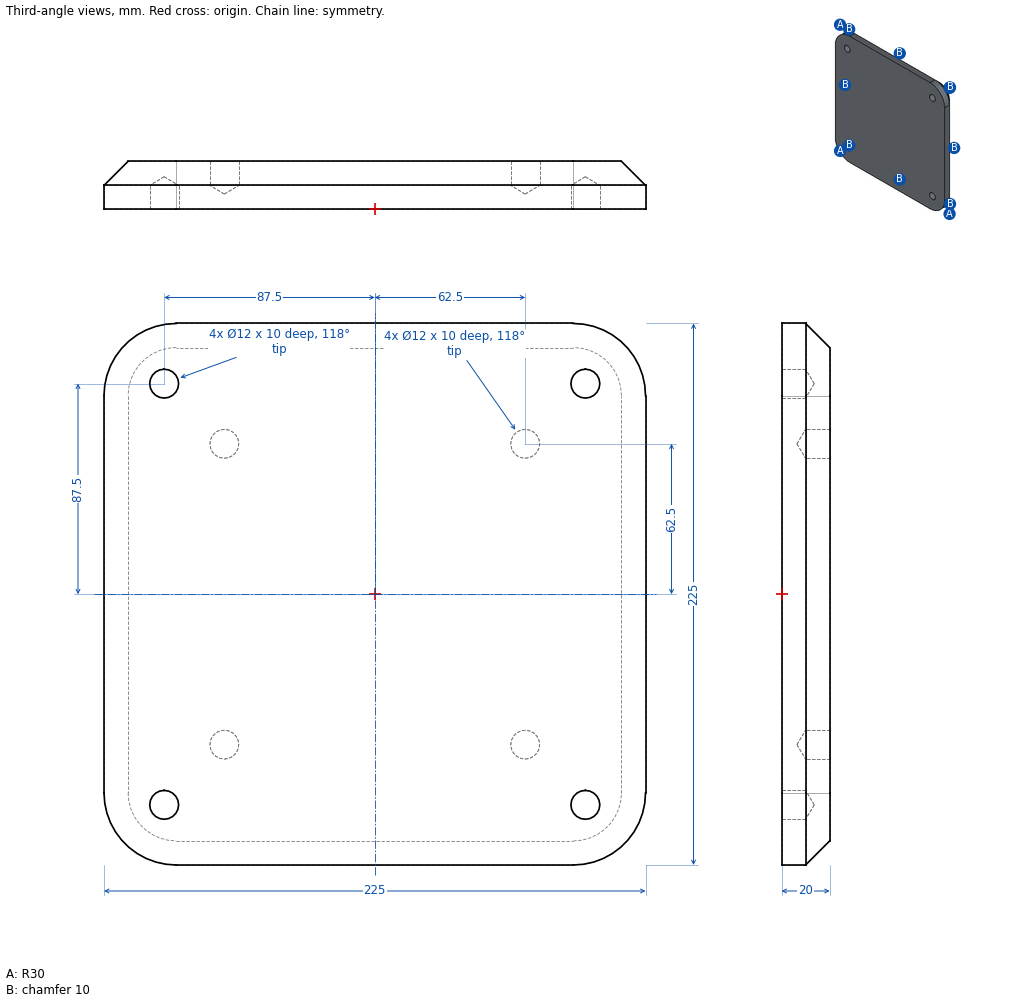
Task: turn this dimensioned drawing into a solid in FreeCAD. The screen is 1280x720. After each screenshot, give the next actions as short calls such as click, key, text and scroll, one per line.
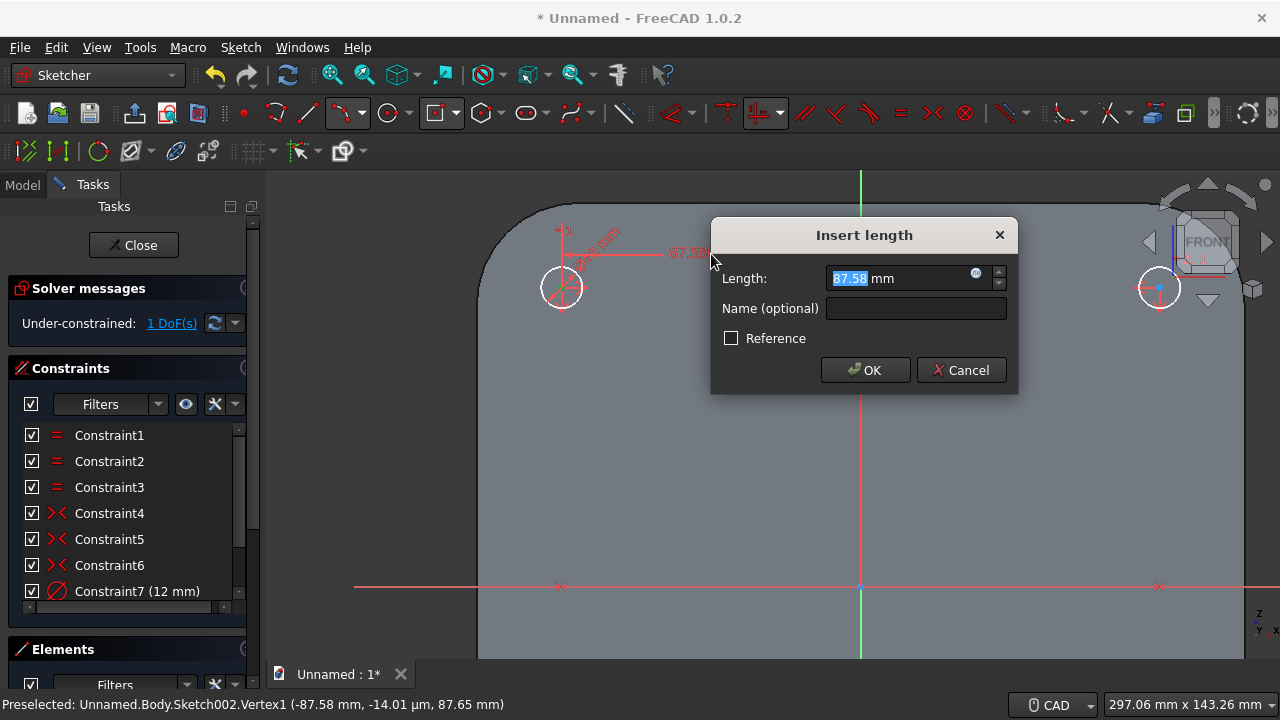
text(87.5)
key(Return)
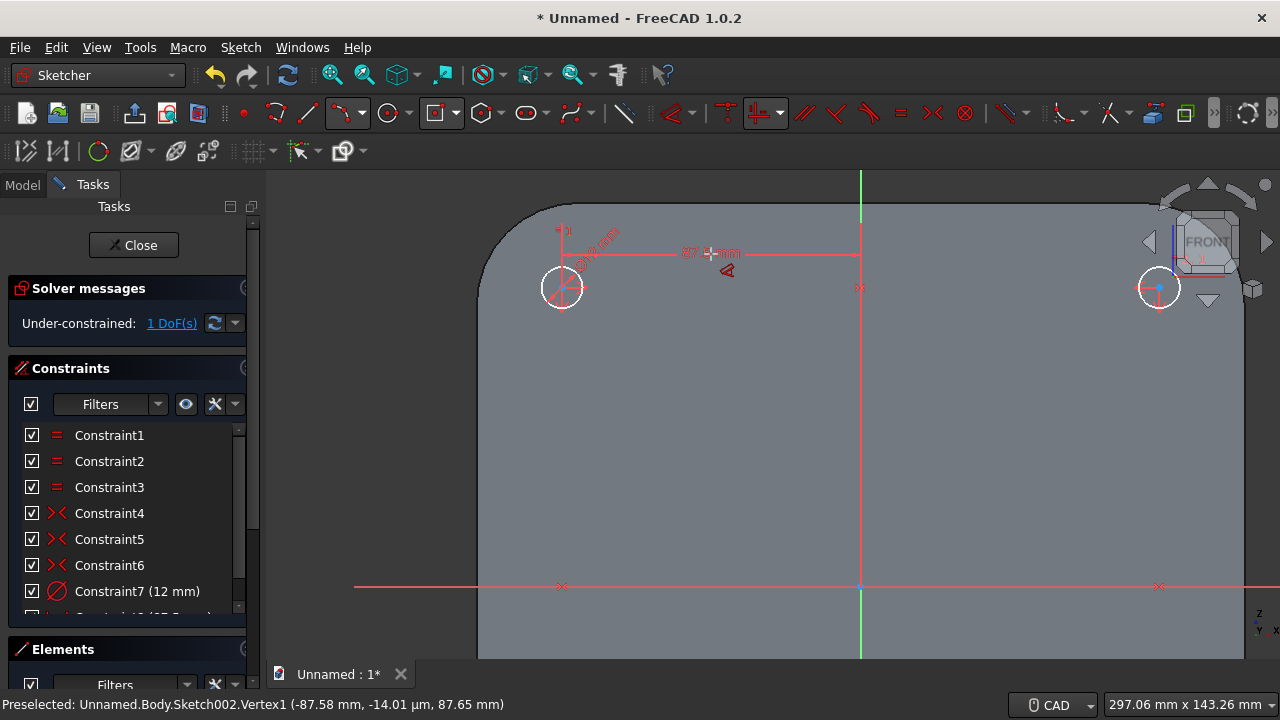
click(562, 288)
click(528, 437)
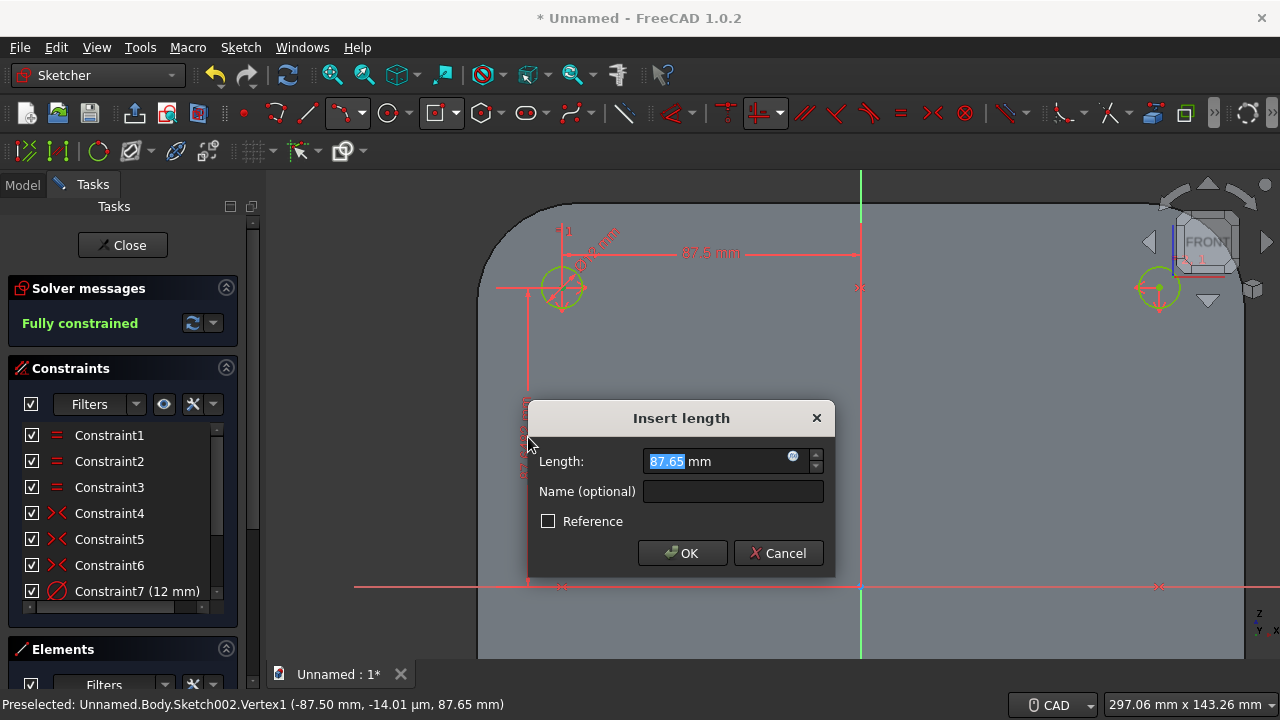
text(87.5)
key(Return)
key(Escape)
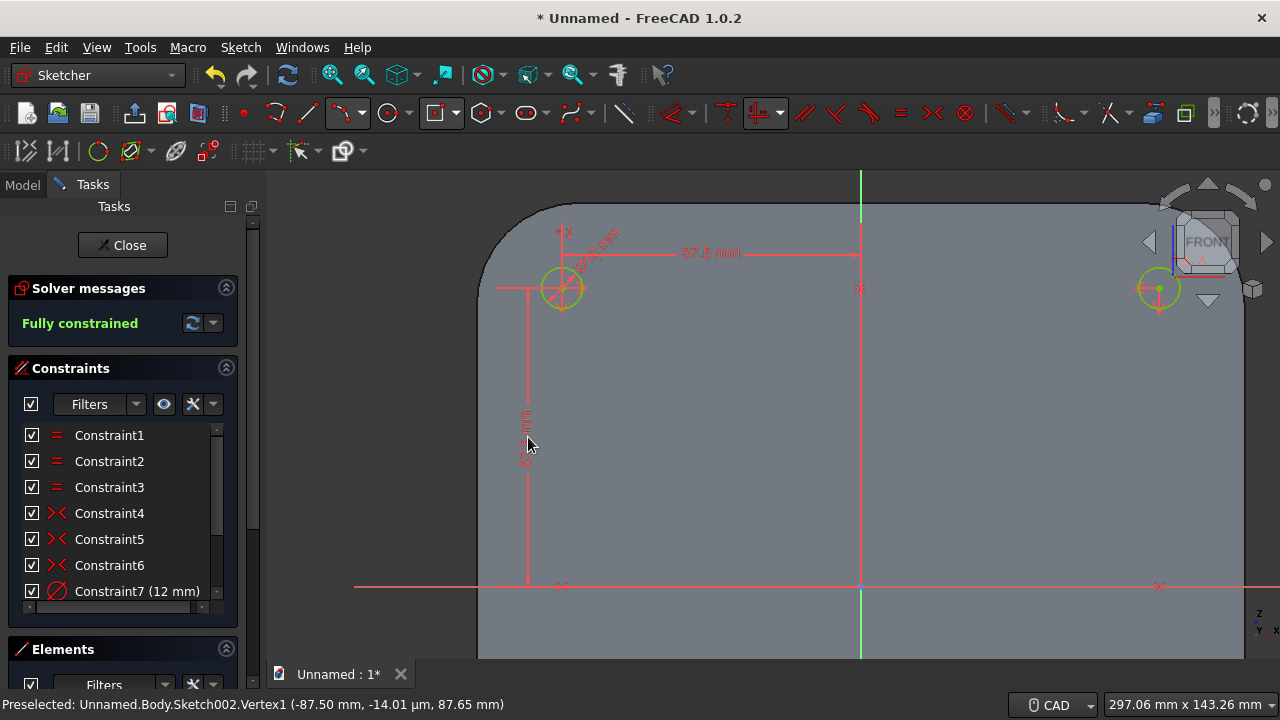
click(123, 245)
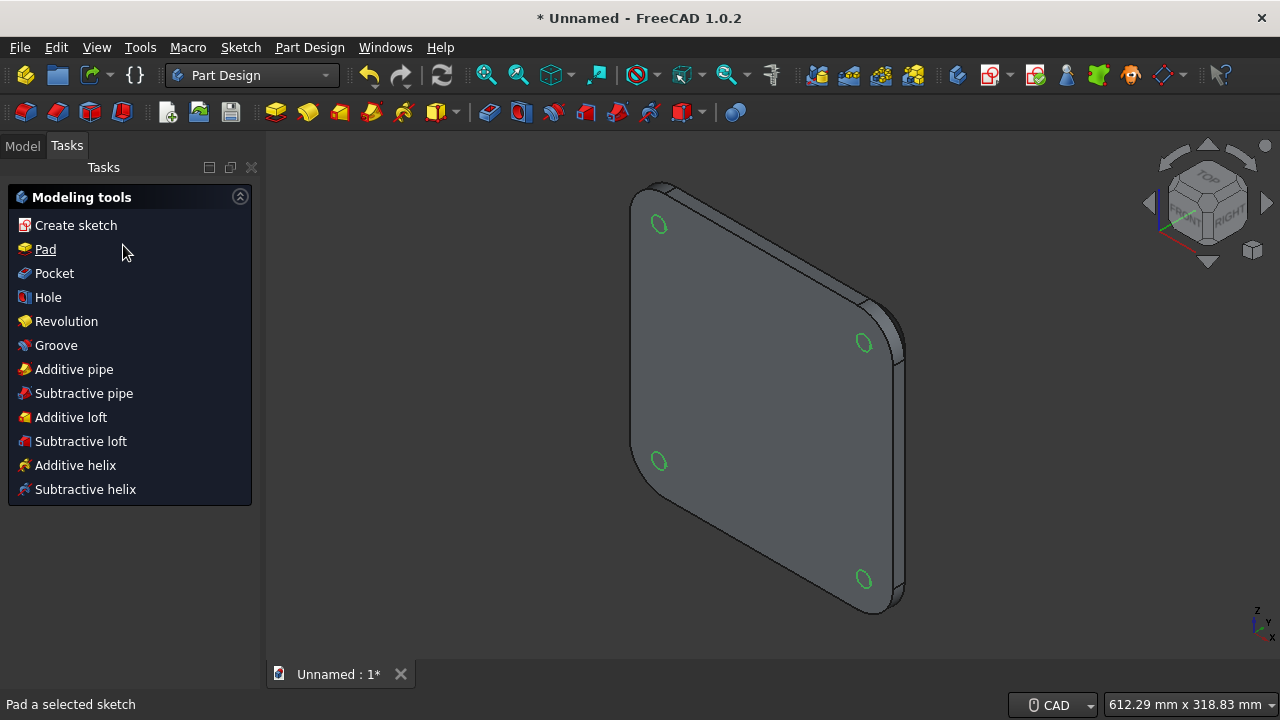
click(522, 112)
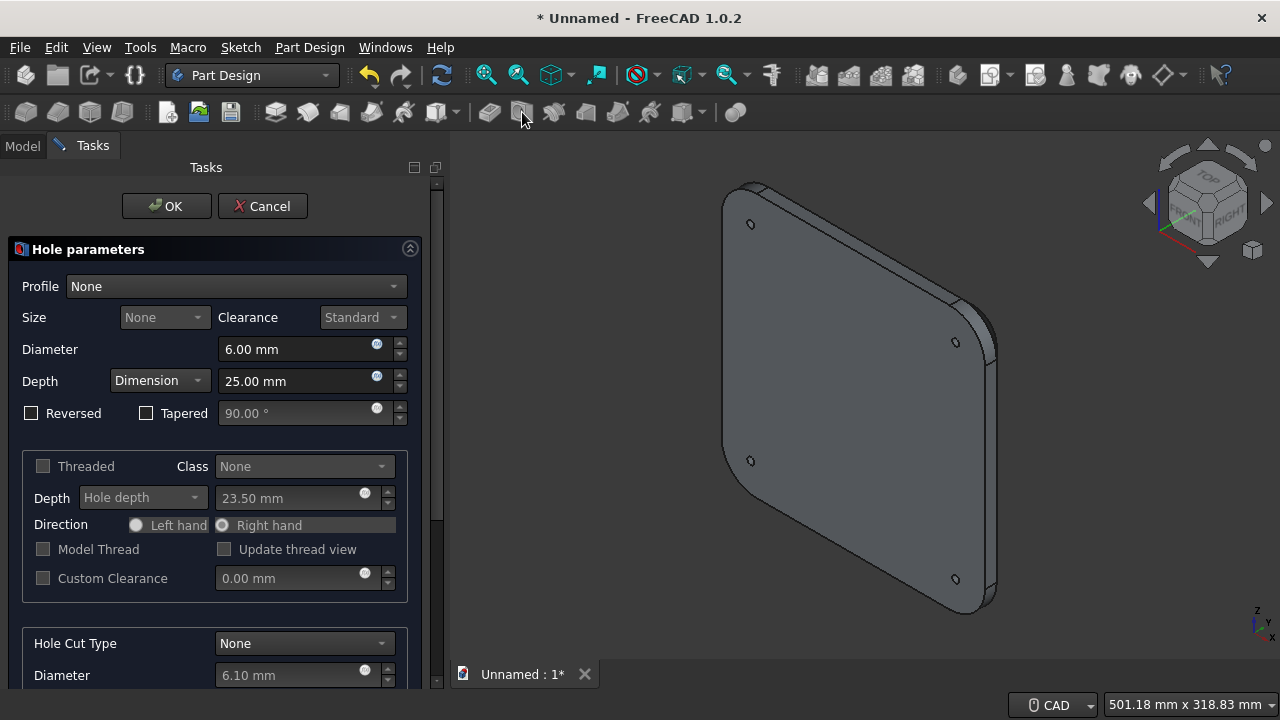
triple_click(305, 349)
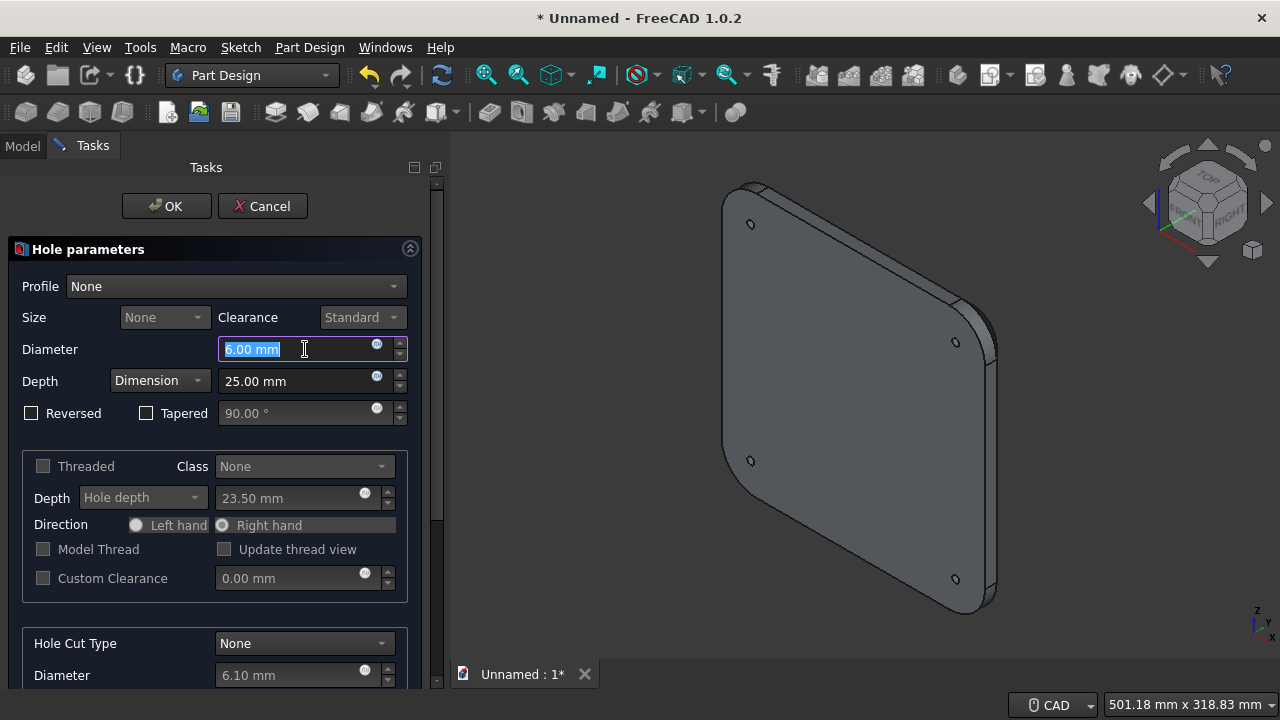
text(12)
key(Tab)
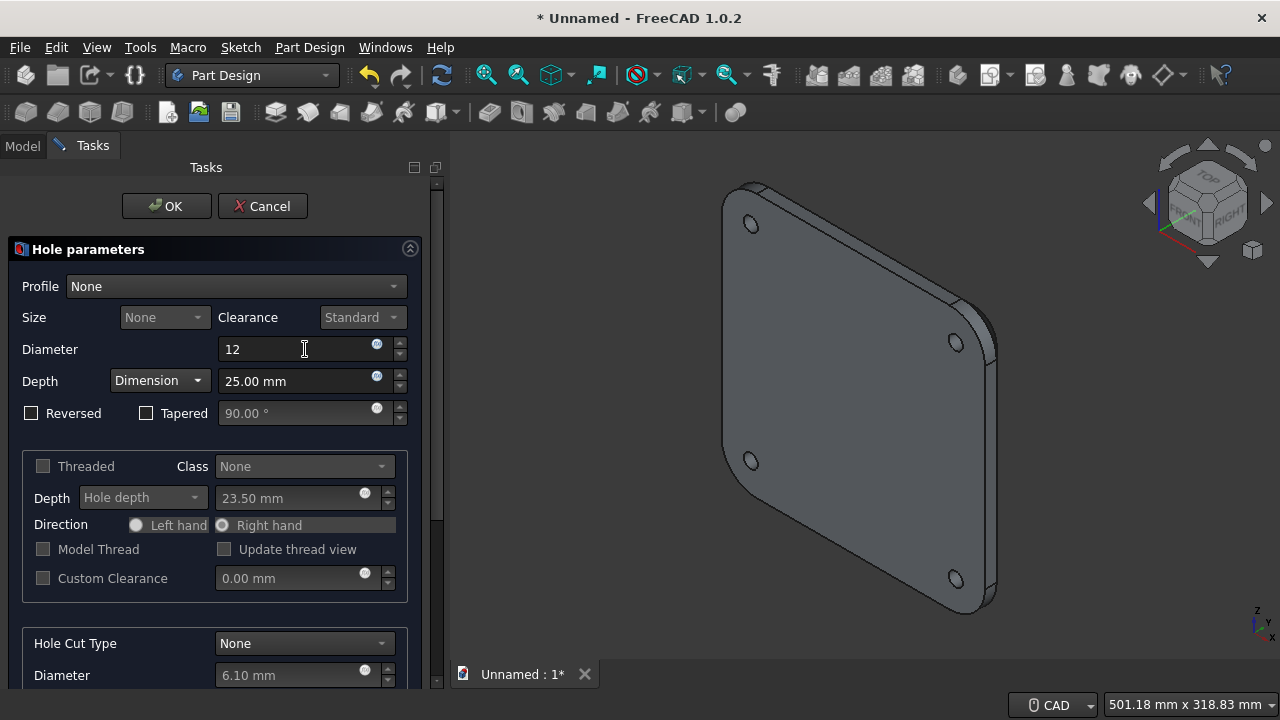
triple_click(305, 381)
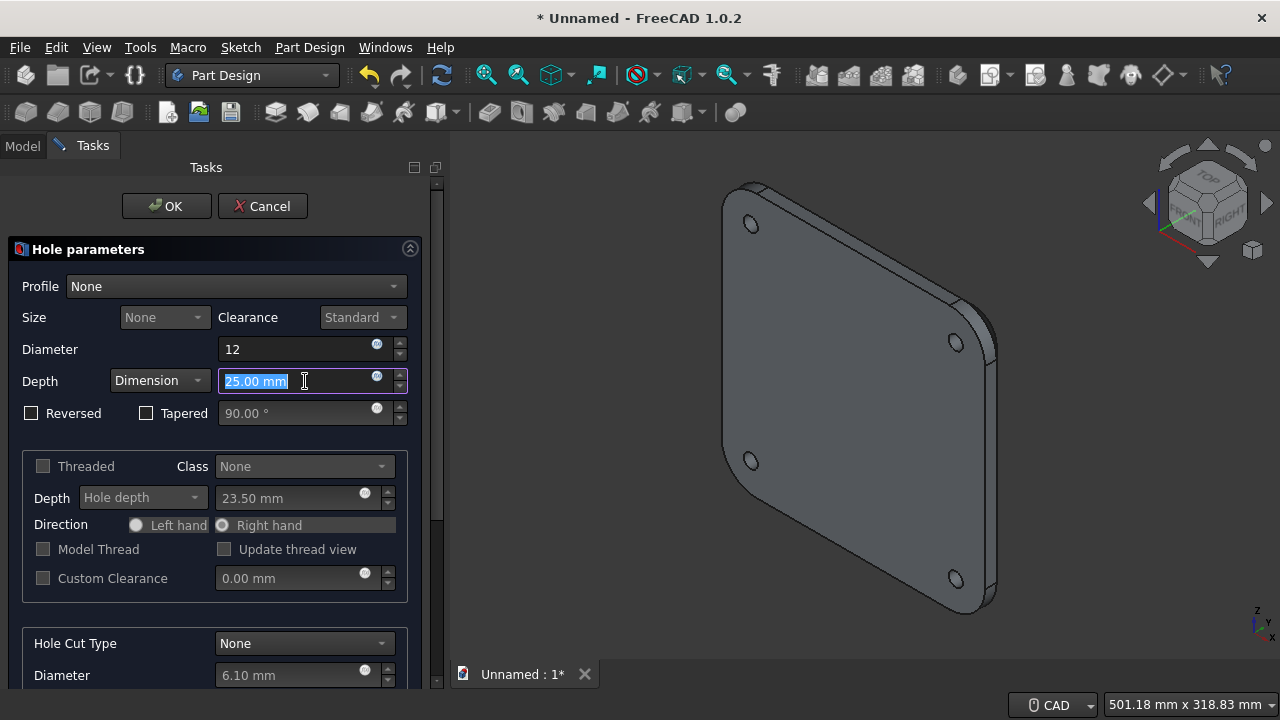
text(10)
key(Tab)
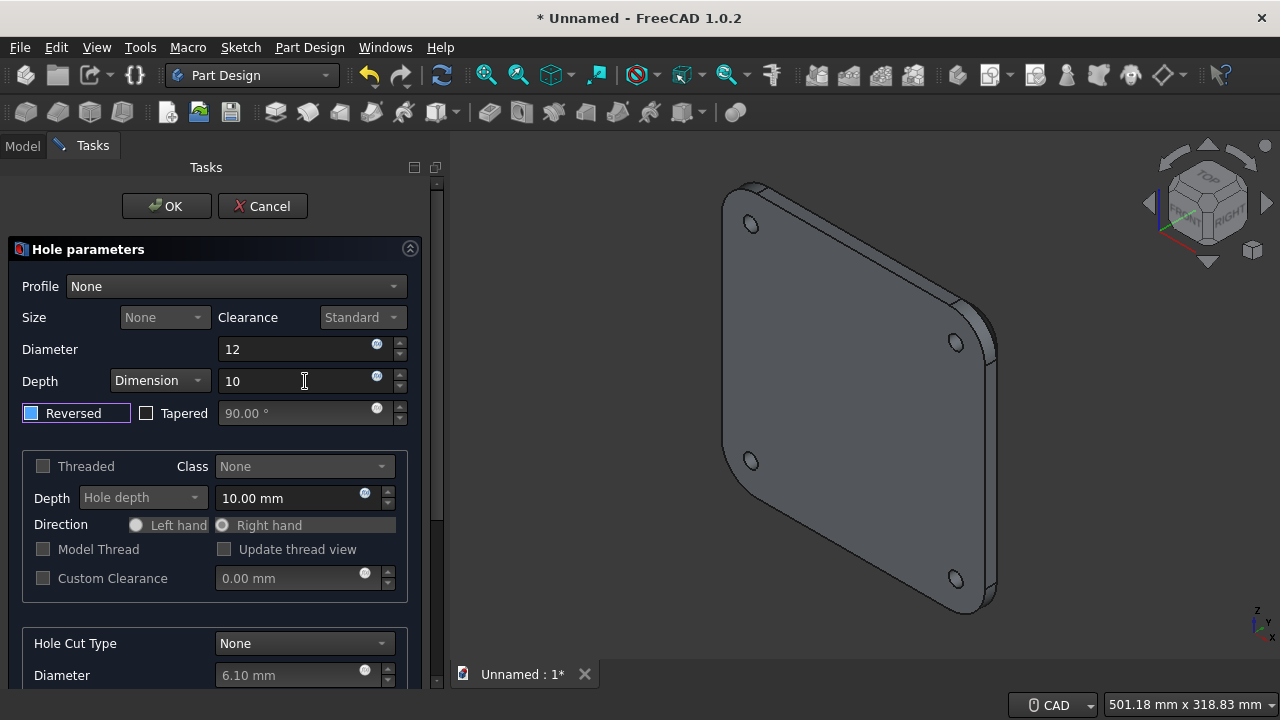
click(167, 206)